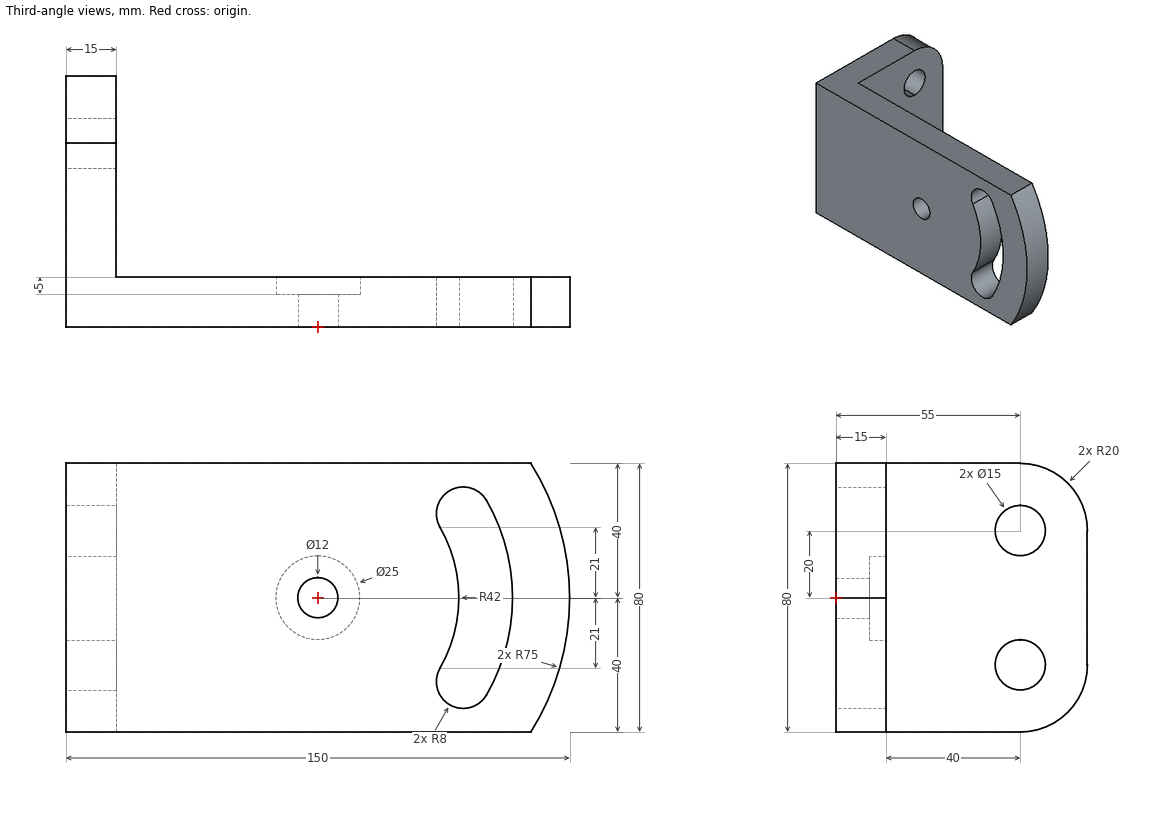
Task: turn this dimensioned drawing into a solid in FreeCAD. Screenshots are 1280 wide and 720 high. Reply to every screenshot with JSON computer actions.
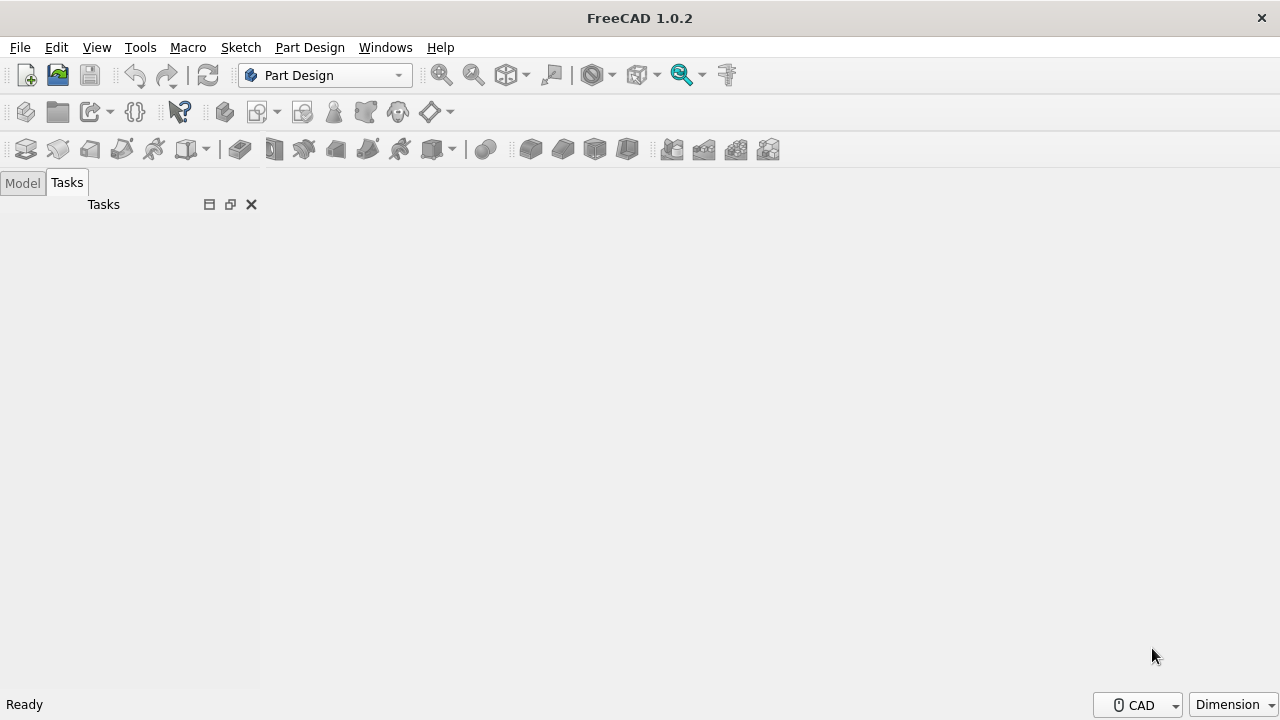
{"action": "left_click", "coordinate": [26, 76]}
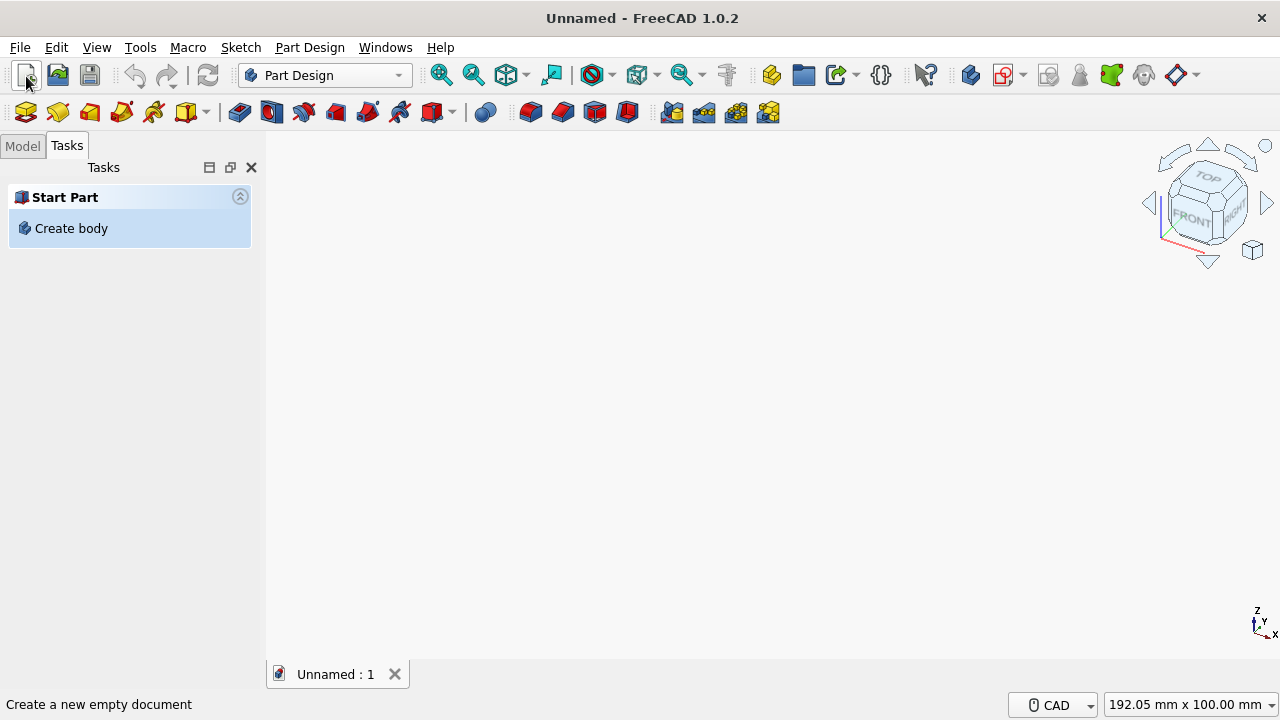
{"action": "left_click", "coordinate": [1004, 76]}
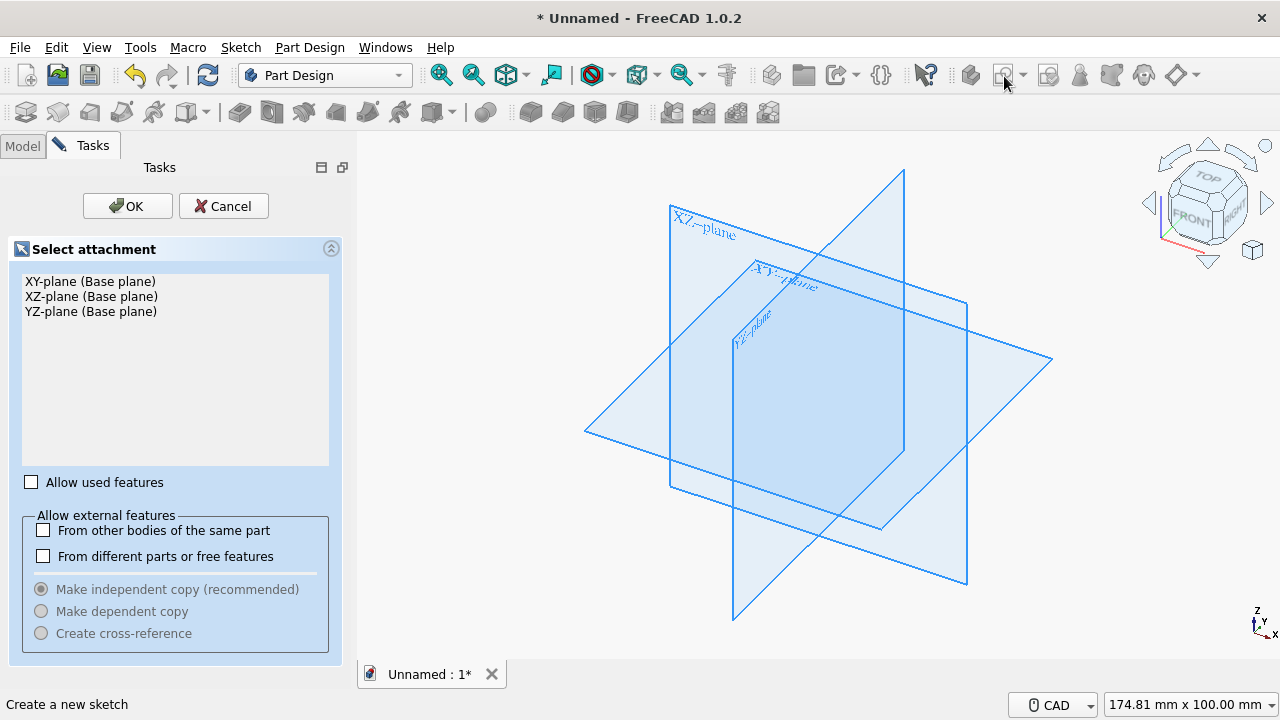
{"action": "left_click", "coordinate": [82, 296]}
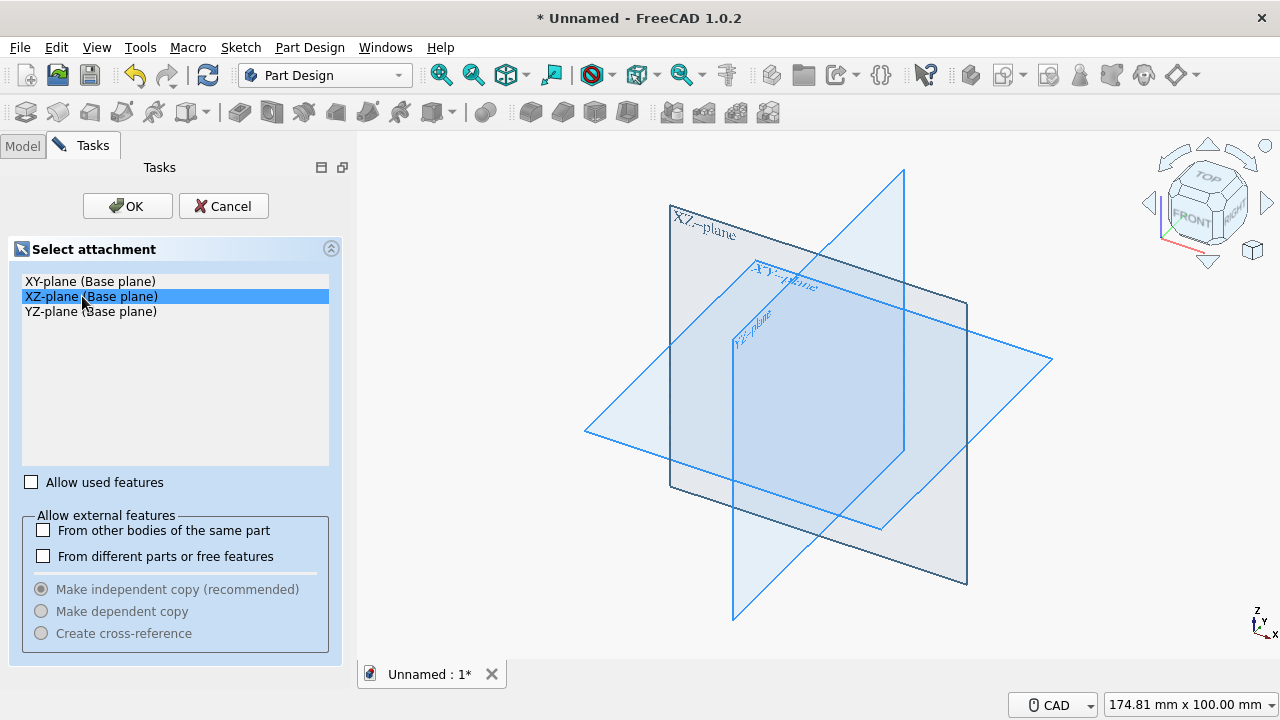
{"action": "left_click", "coordinate": [128, 206]}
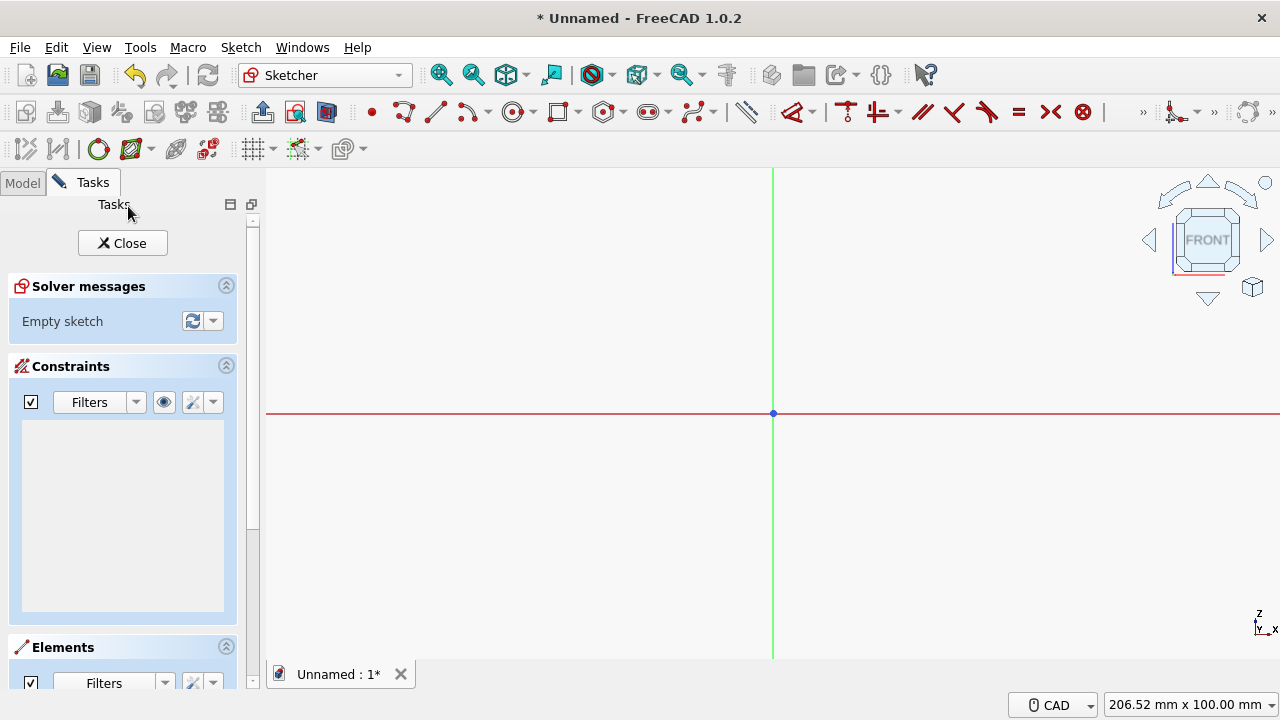
{"action": "scroll", "coordinate": [395, 413], "scroll_direction": "down", "scroll_amount": 1}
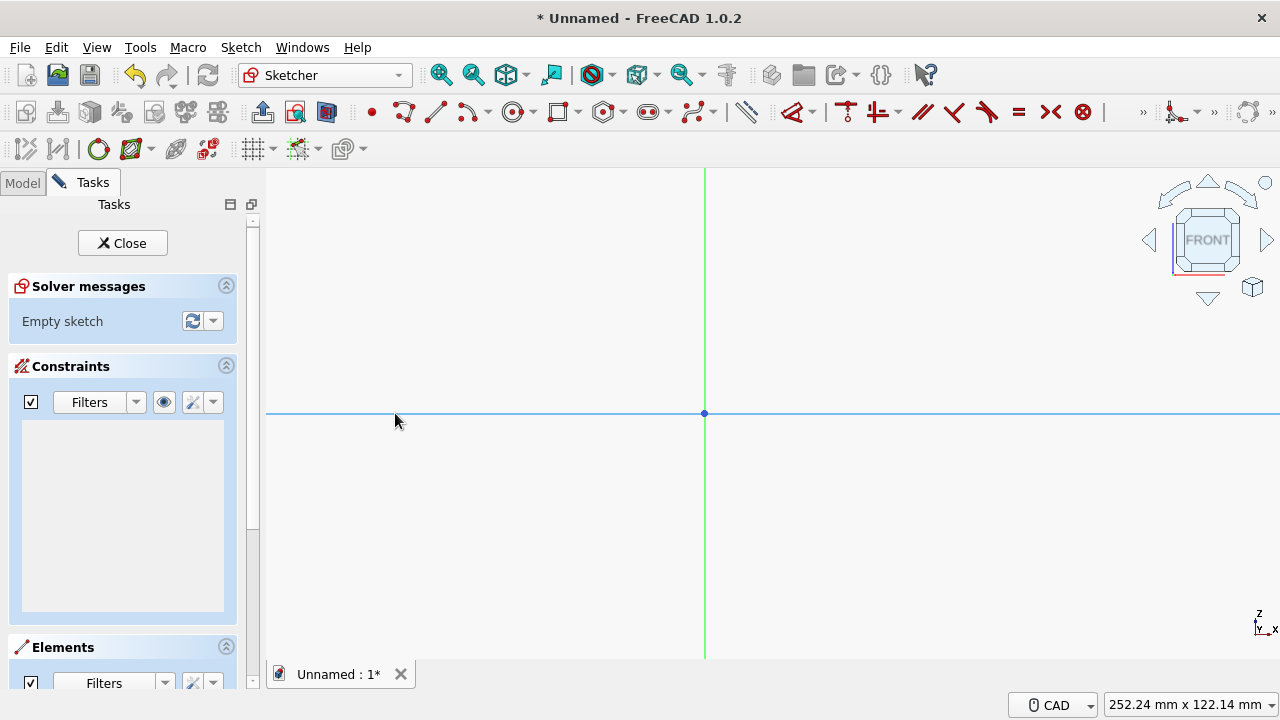
{"action": "left_click", "coordinate": [580, 112]}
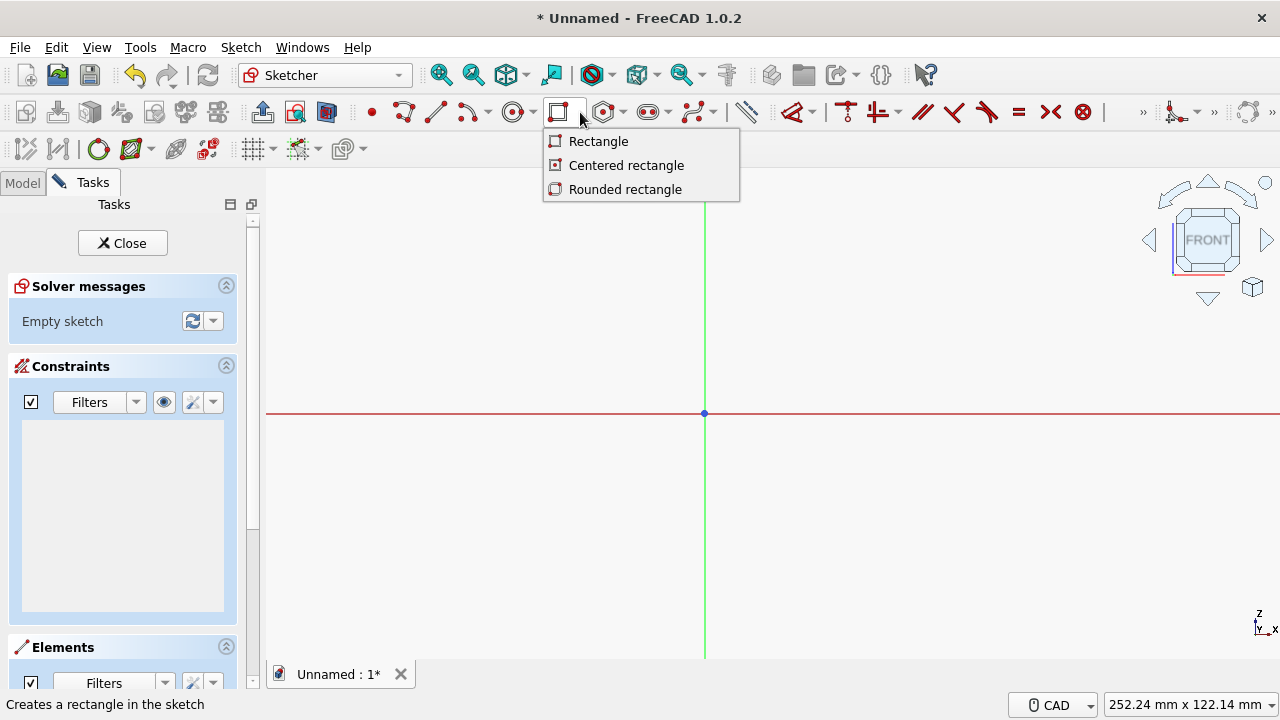
{"action": "left_click", "coordinate": [642, 165]}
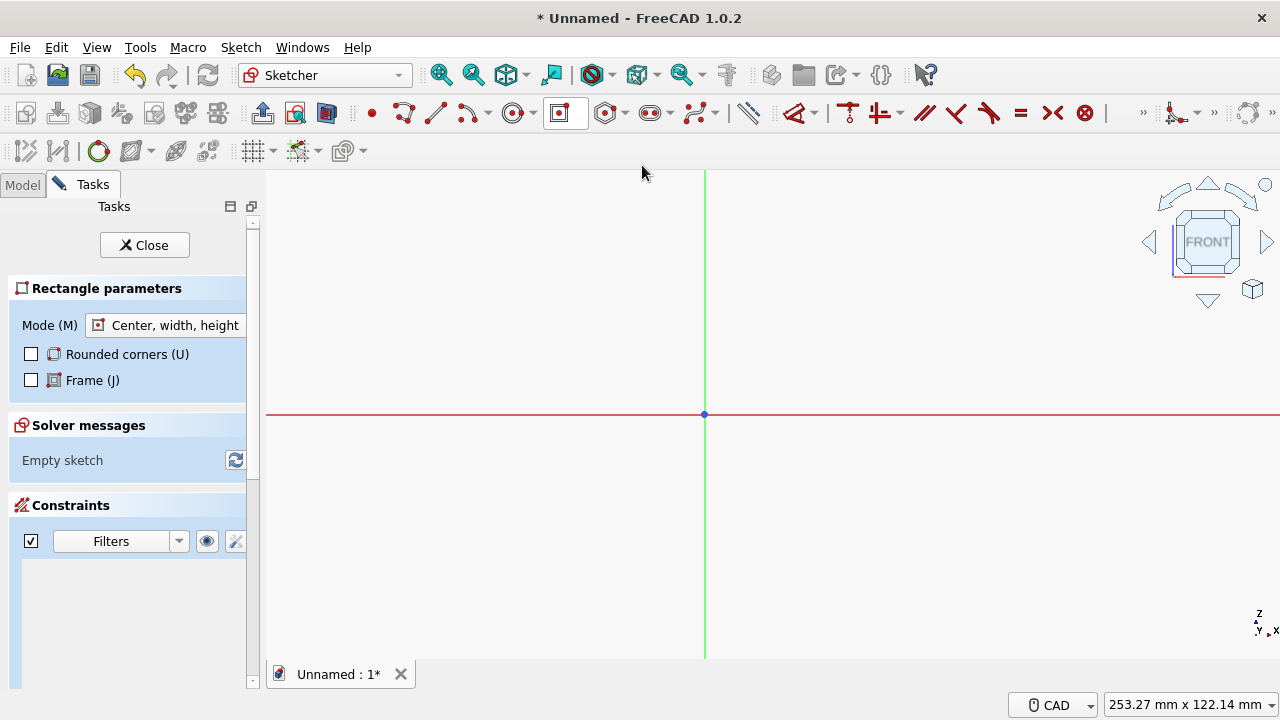
{"action": "left_click", "coordinate": [705, 414]}
{"action": "left_click", "coordinate": [1005, 254]}
{"action": "key", "text": "Escape"}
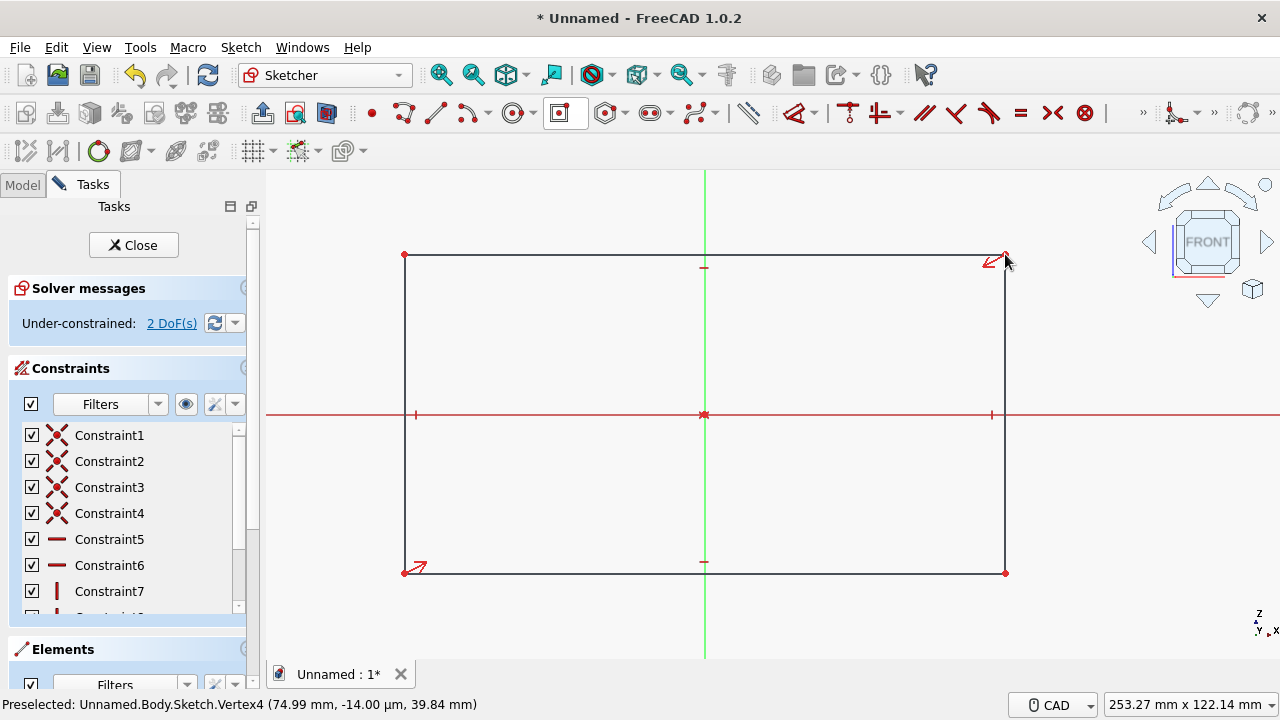
{"action": "key", "text": "d"}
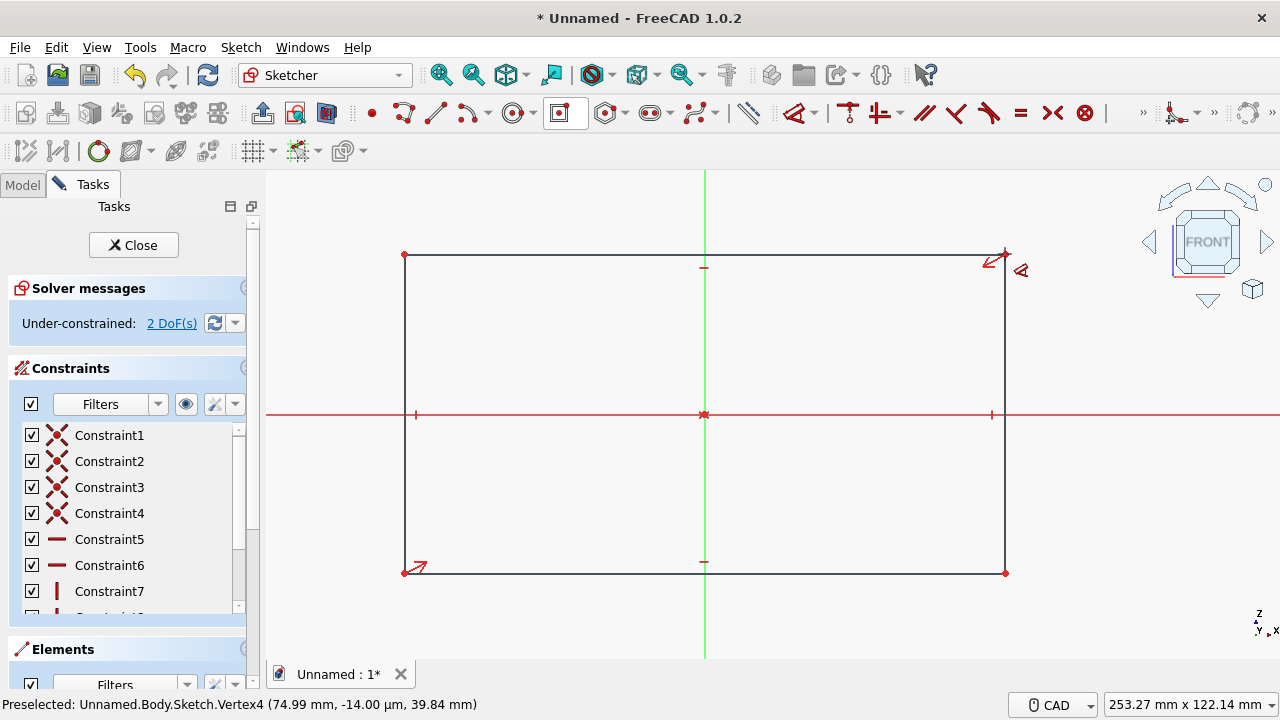
{"action": "left_click", "coordinate": [1005, 478]}
{"action": "left_click", "coordinate": [1039, 341]}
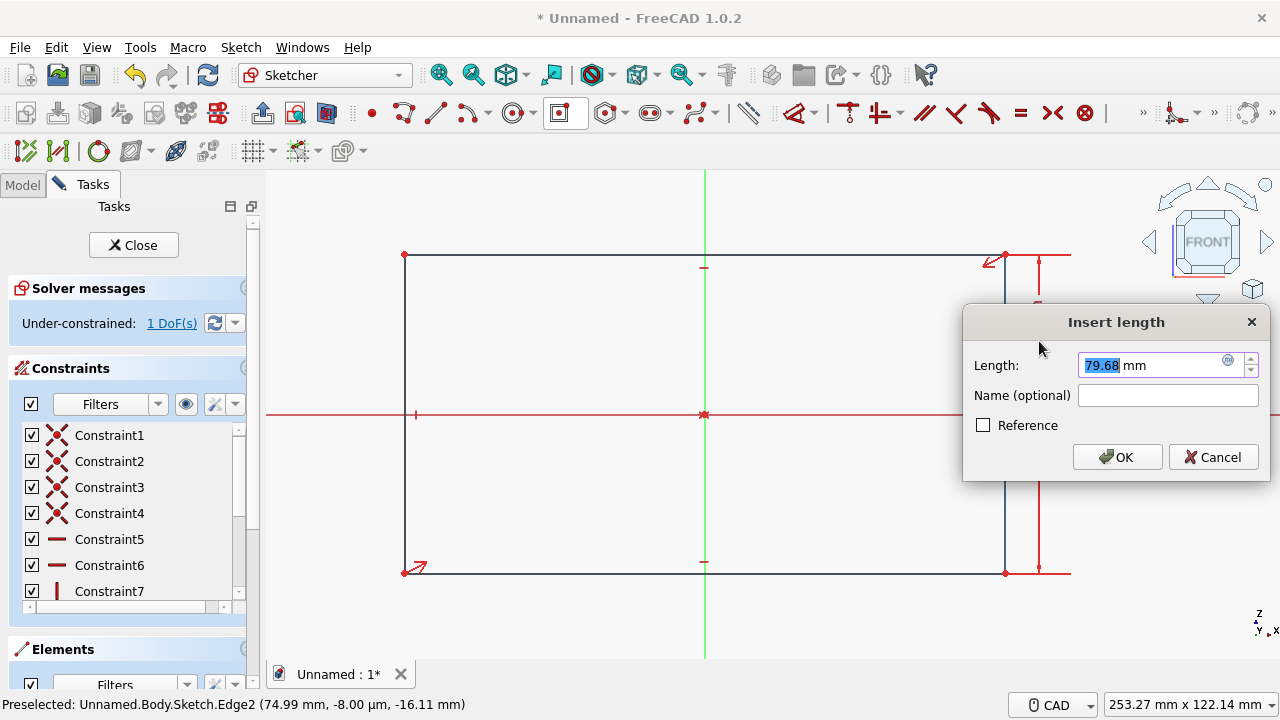
{"action": "type", "text": "80"}
{"action": "key", "text": "Return"}